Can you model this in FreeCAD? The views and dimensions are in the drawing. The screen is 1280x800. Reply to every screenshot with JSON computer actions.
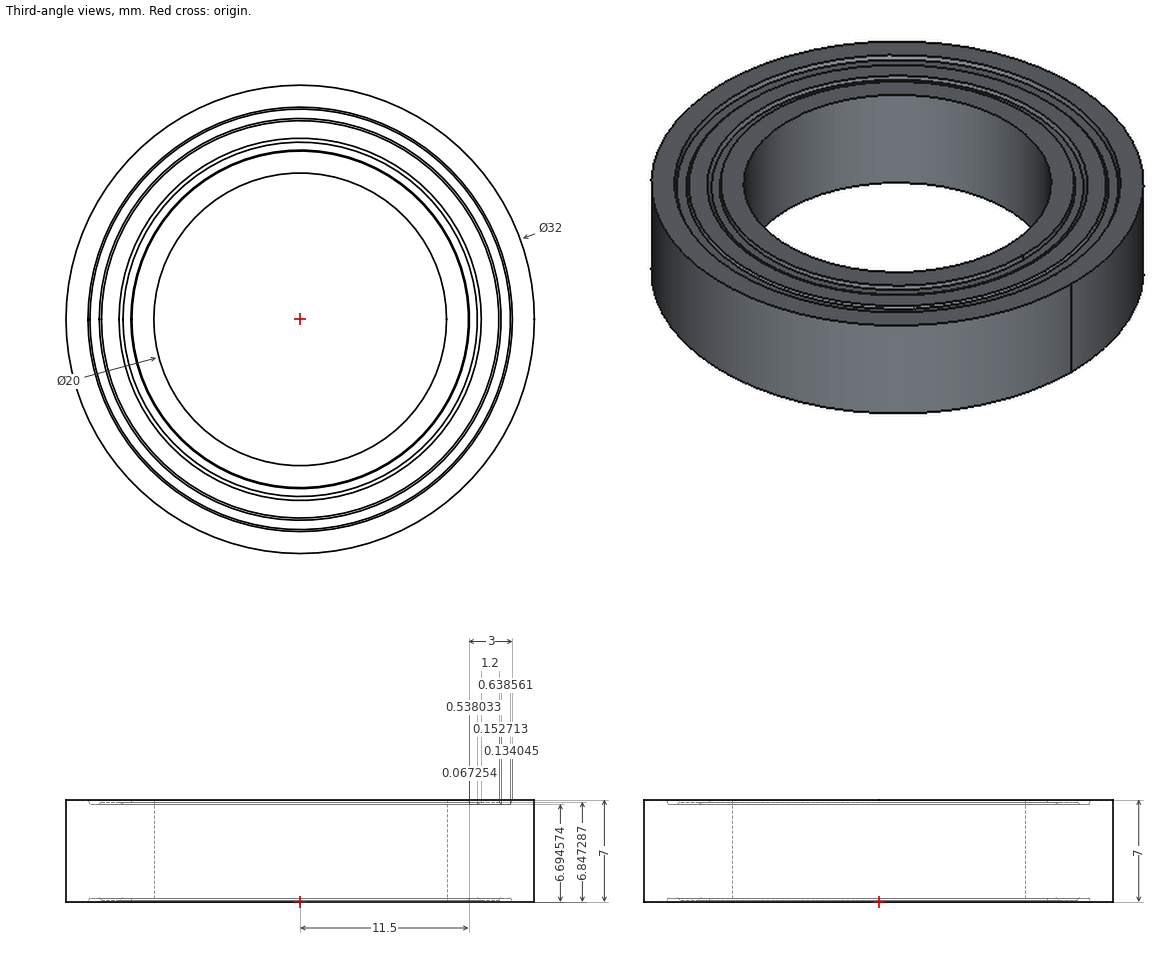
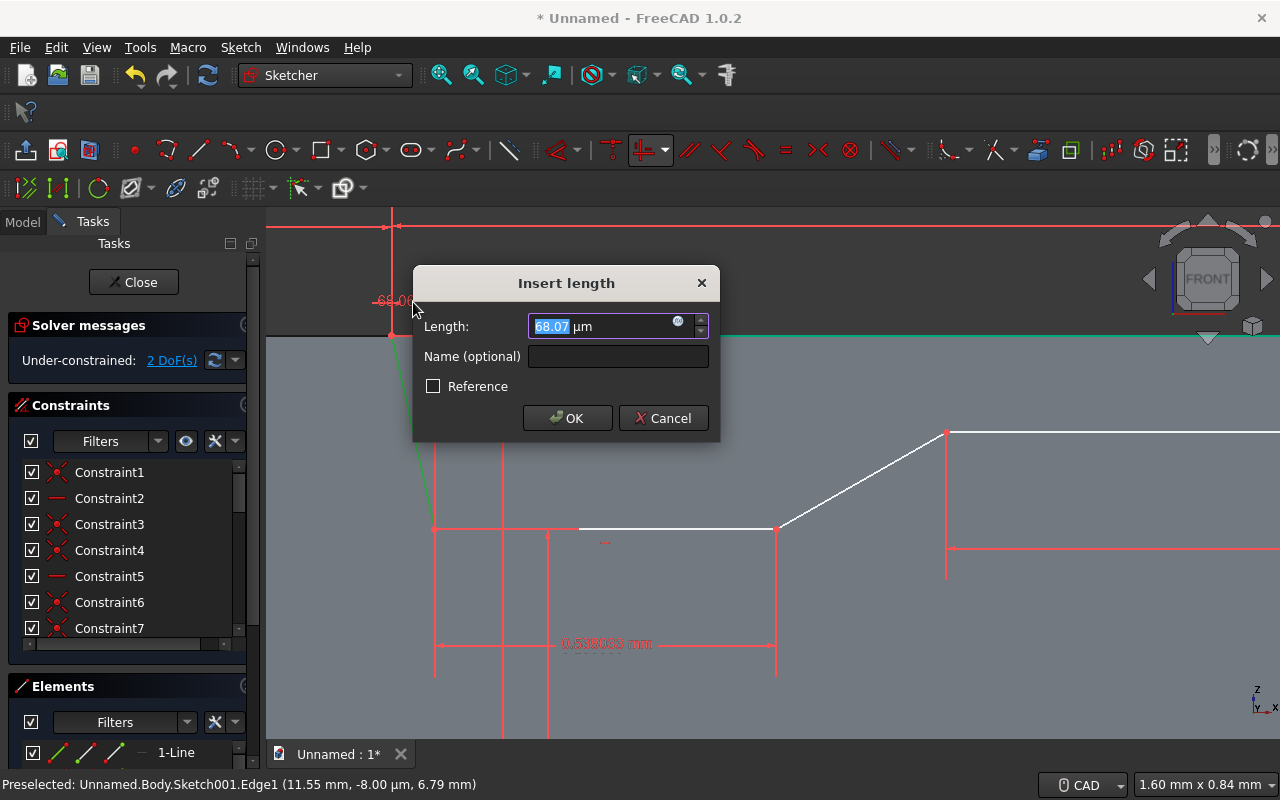
{"action": "key", "text": "ctrl+a"}
{"action": "type", "text": "0.067254 mm"}
{"action": "key", "text": "Return"}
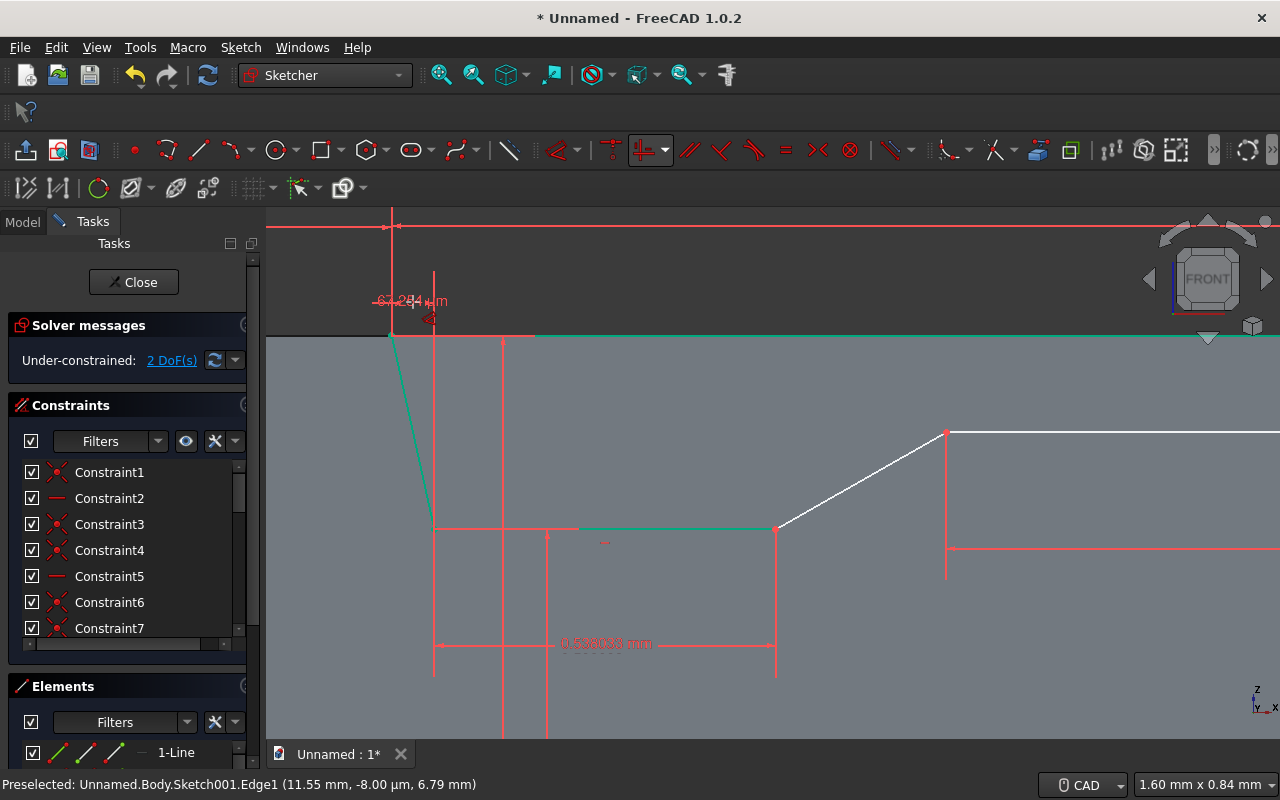
{"action": "scroll", "coordinate": [429, 490], "scroll_direction": "down", "scroll_amount": 6}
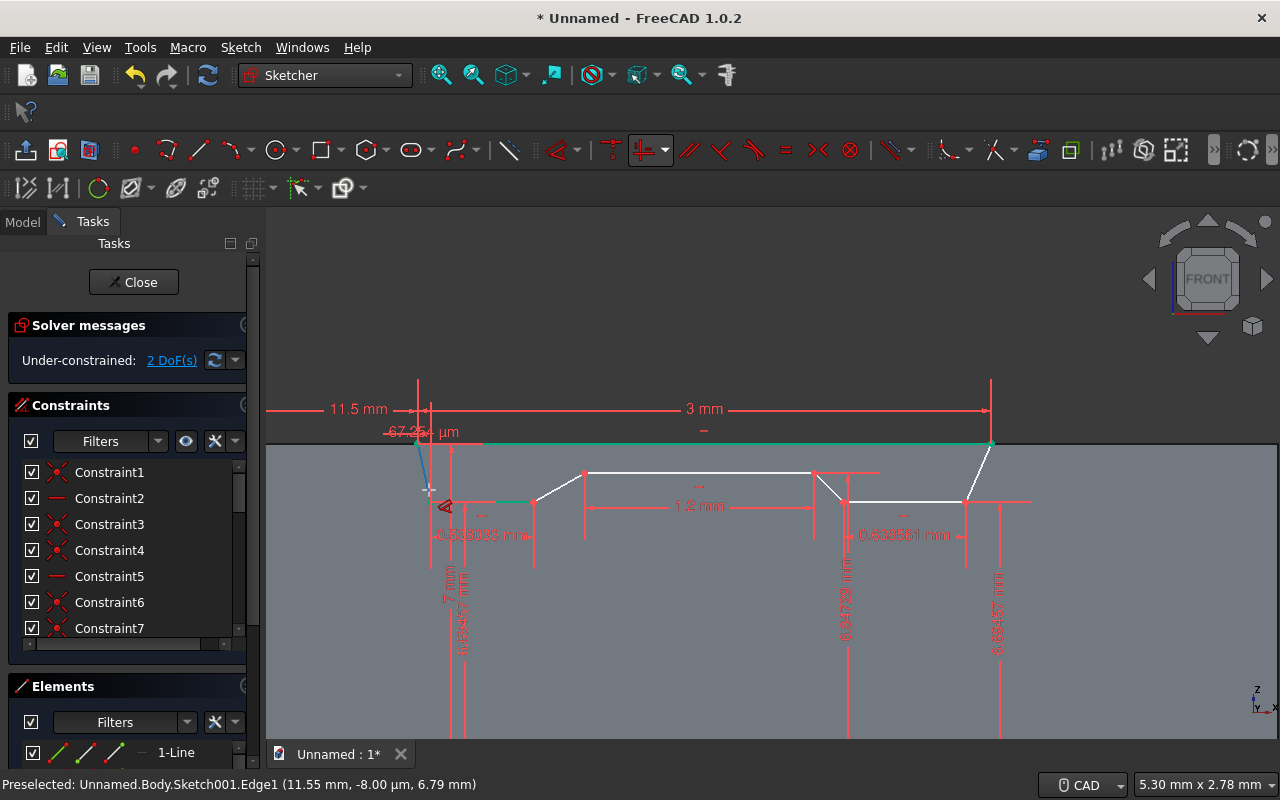
{"action": "scroll", "coordinate": [984, 461], "scroll_direction": "up", "scroll_amount": 3}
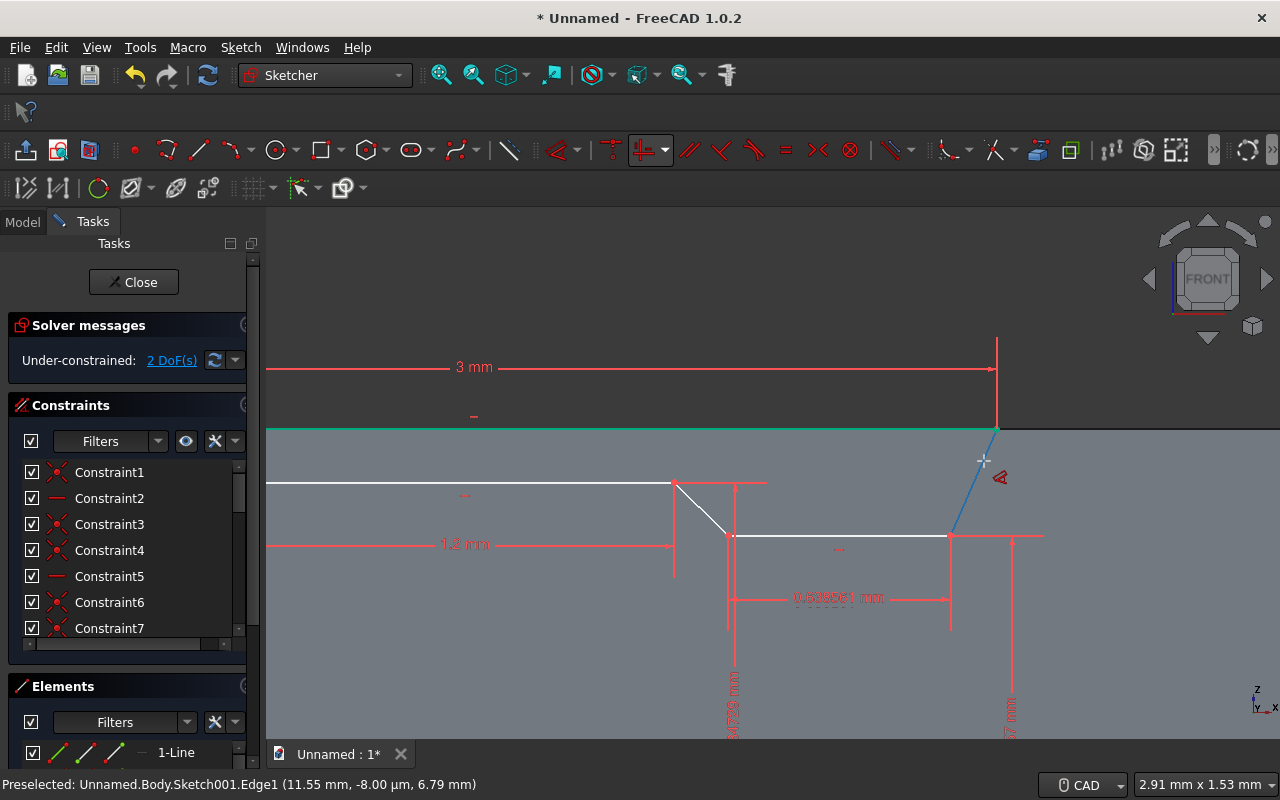
{"action": "left_click", "coordinate": [983, 461]}
{"action": "left_click", "coordinate": [974, 395]}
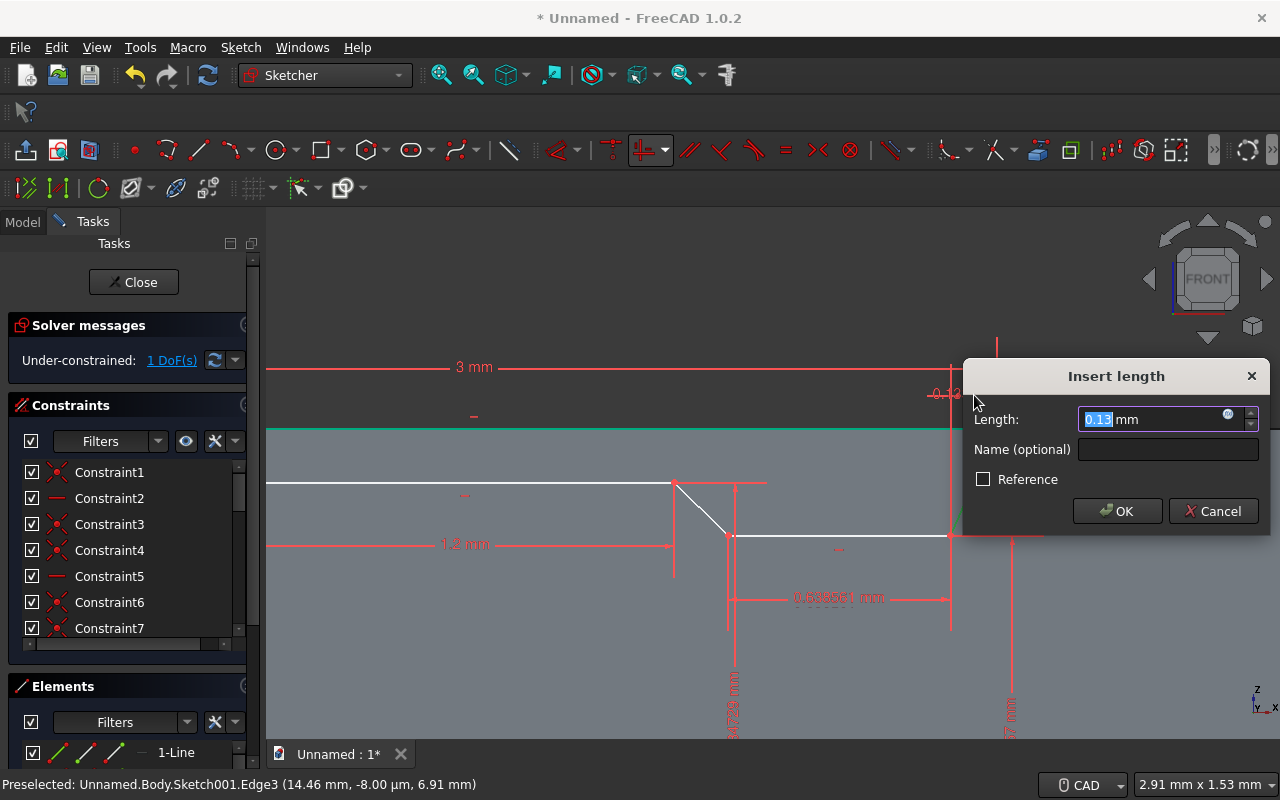
{"action": "type", "text": "0.134045"}
{"action": "key", "text": "Return"}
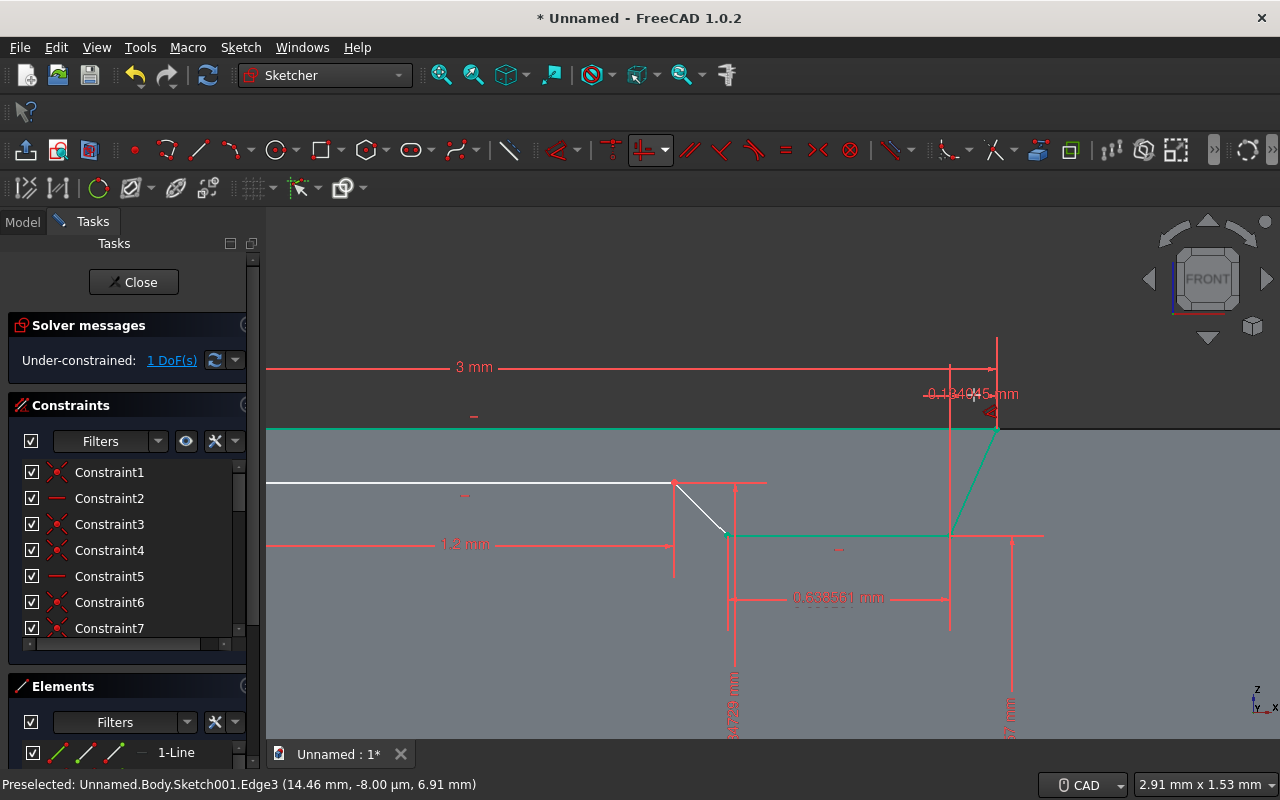
{"action": "left_click", "coordinate": [712, 520]}
{"action": "left_click", "coordinate": [701, 570]}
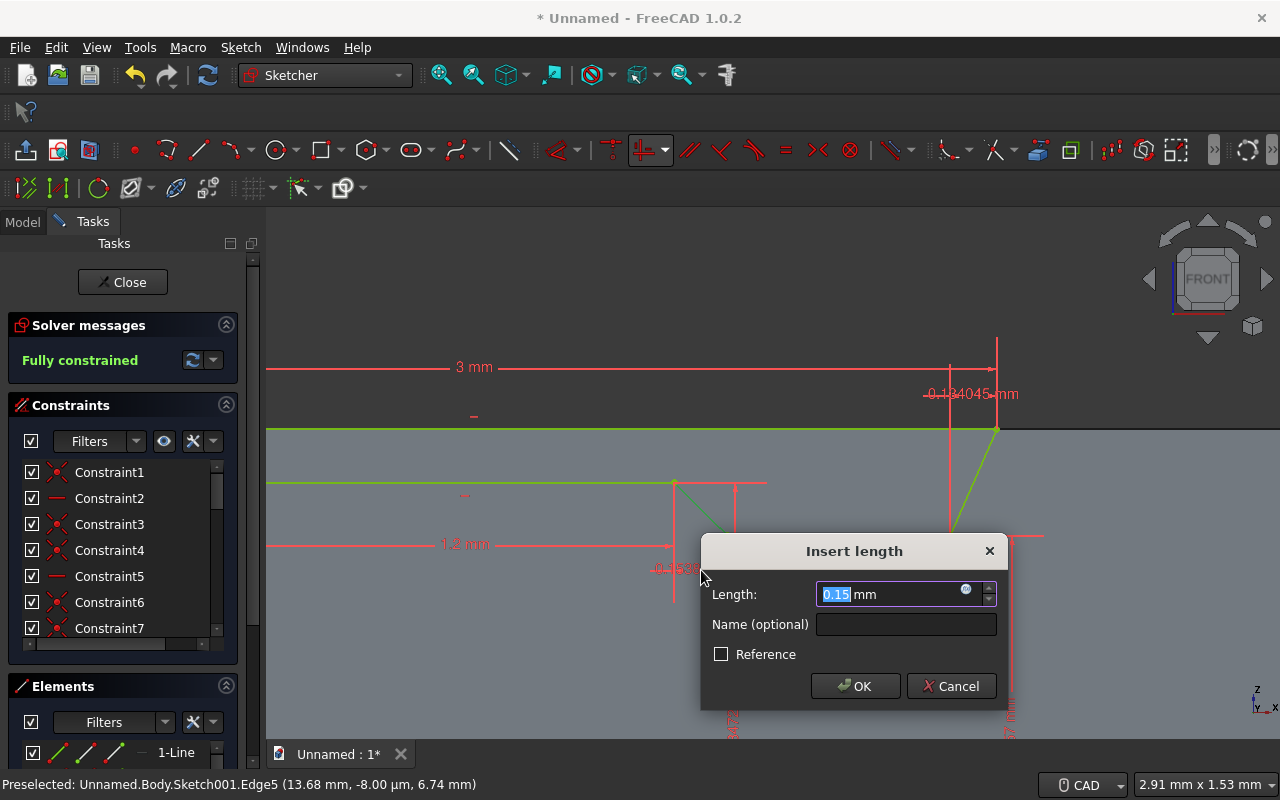
{"action": "type", "text": "0.152713"}
{"action": "key", "text": "Return"}
{"action": "key", "text": "Escape"}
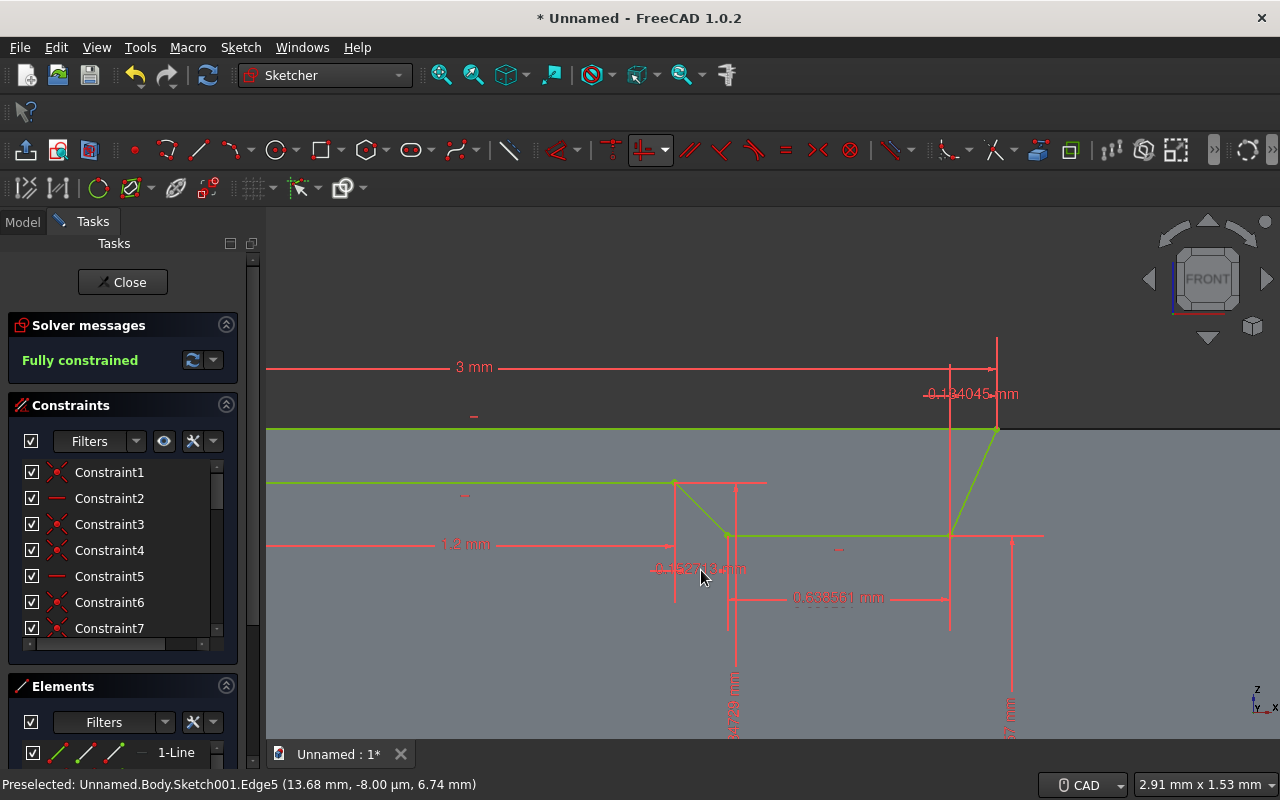
{"action": "left_click", "coordinate": [123, 282]}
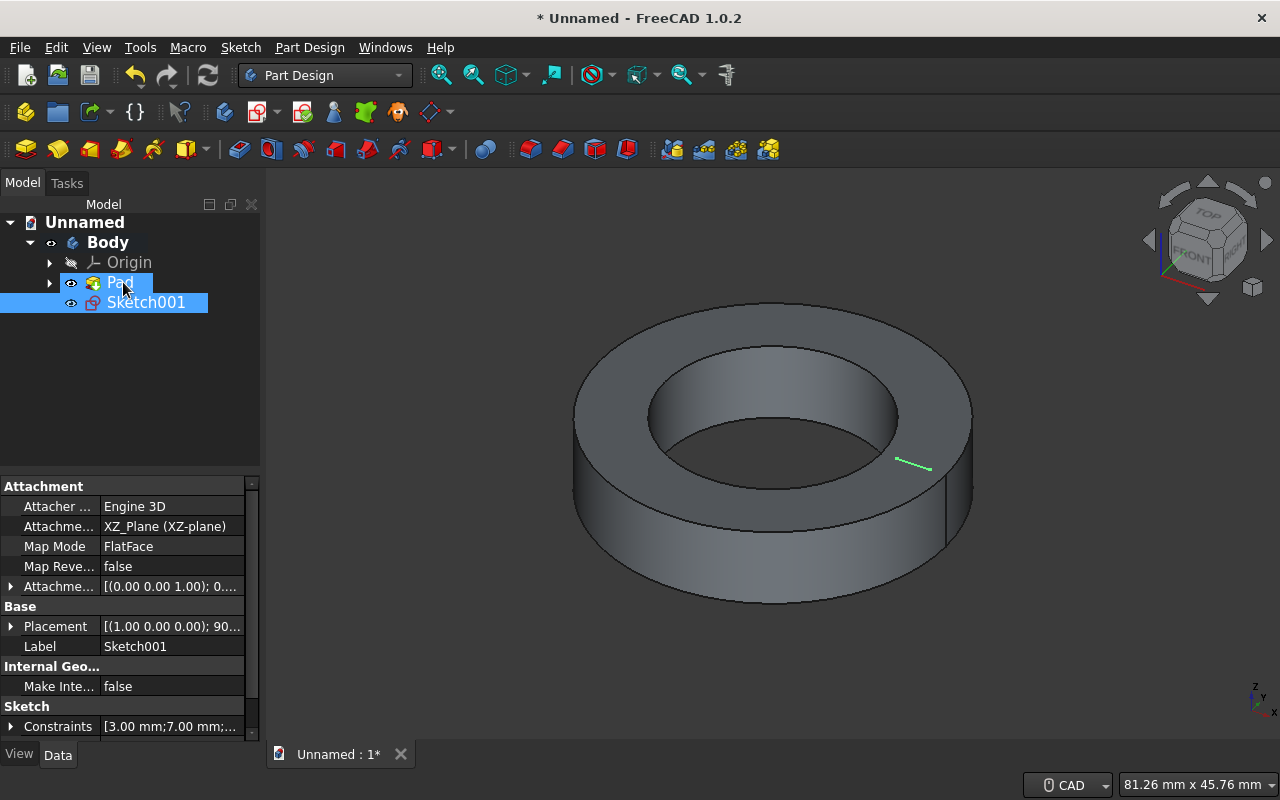
{"action": "left_click", "coordinate": [304, 150]}